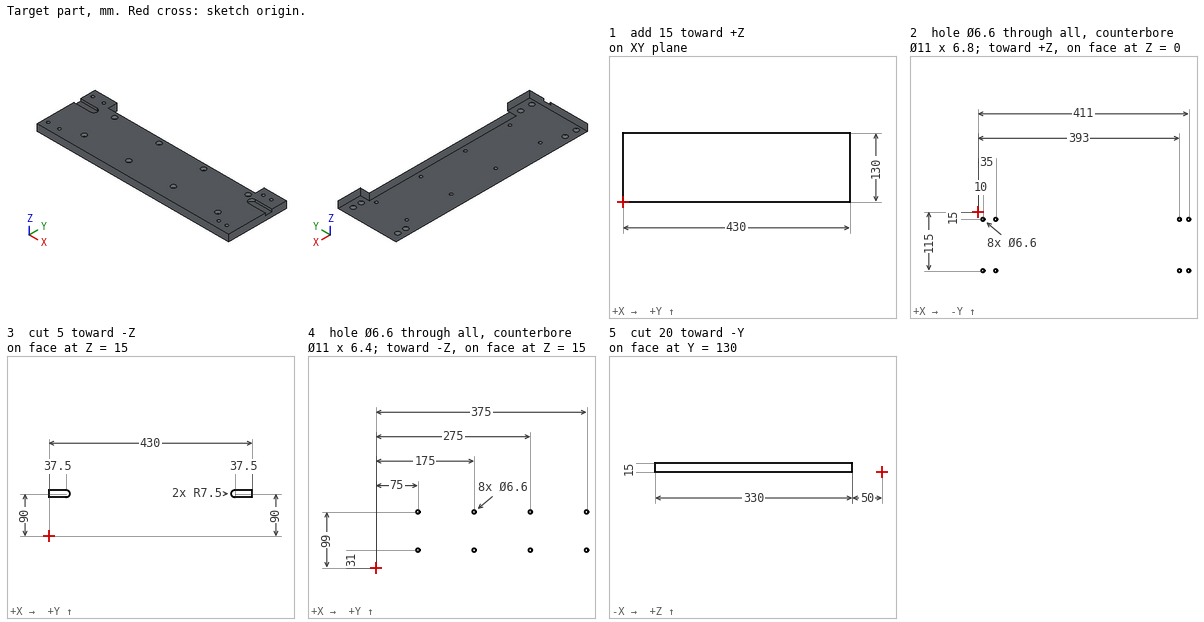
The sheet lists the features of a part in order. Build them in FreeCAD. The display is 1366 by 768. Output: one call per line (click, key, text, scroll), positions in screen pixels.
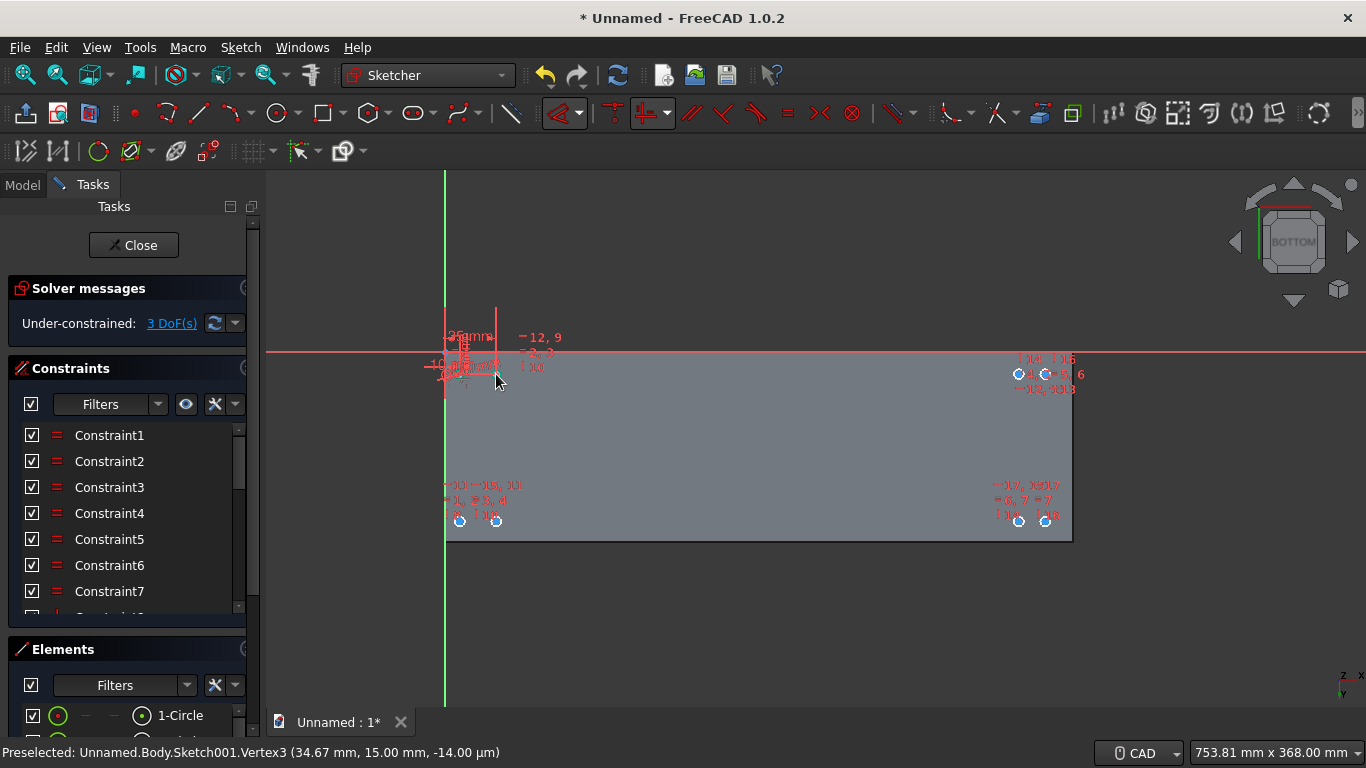
click(460, 522)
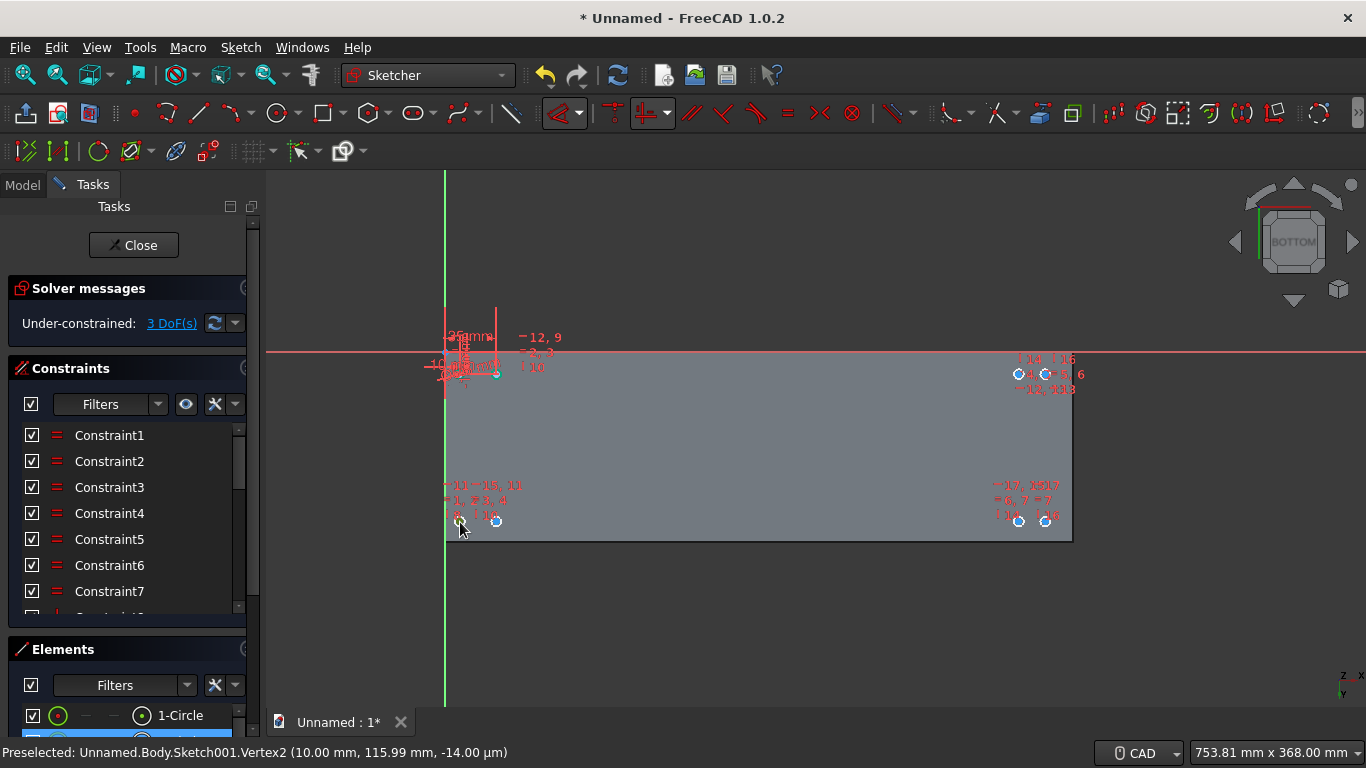
click(582, 114)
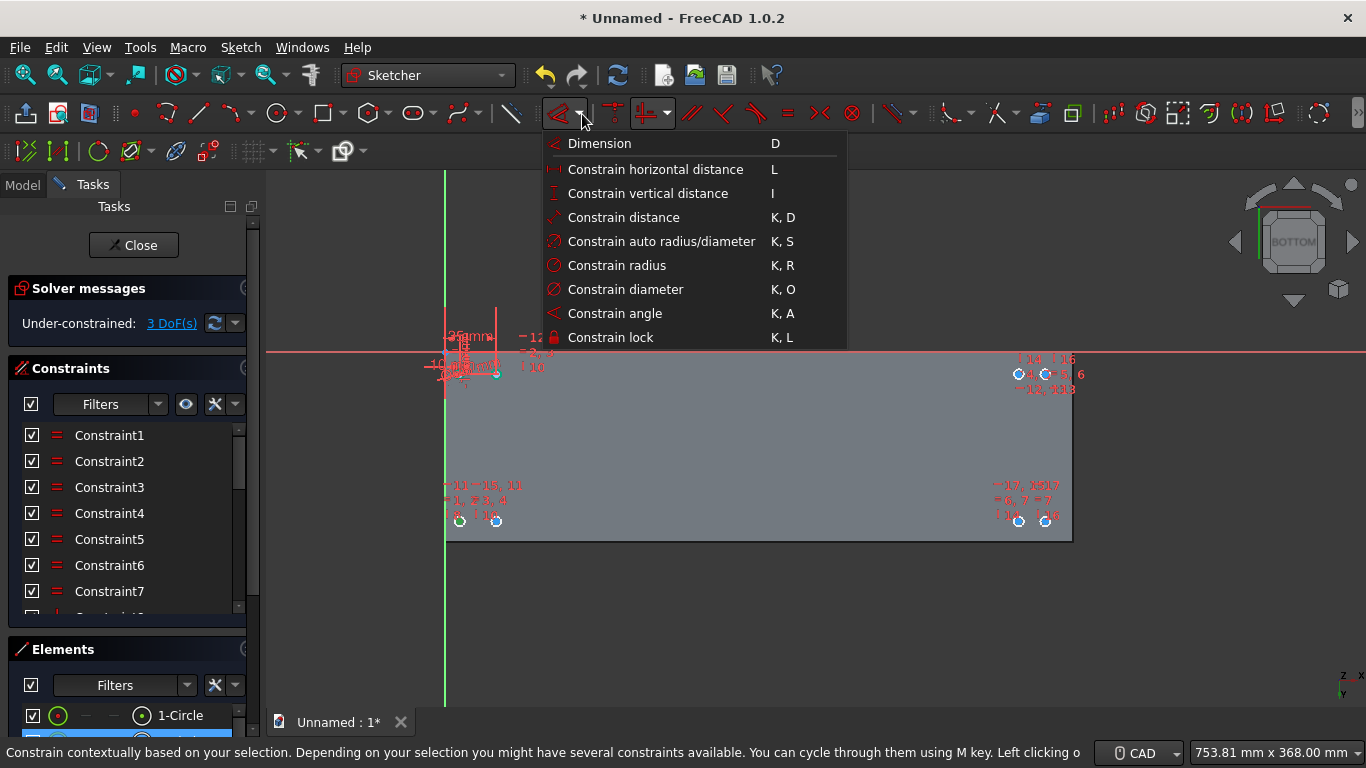
click(695, 193)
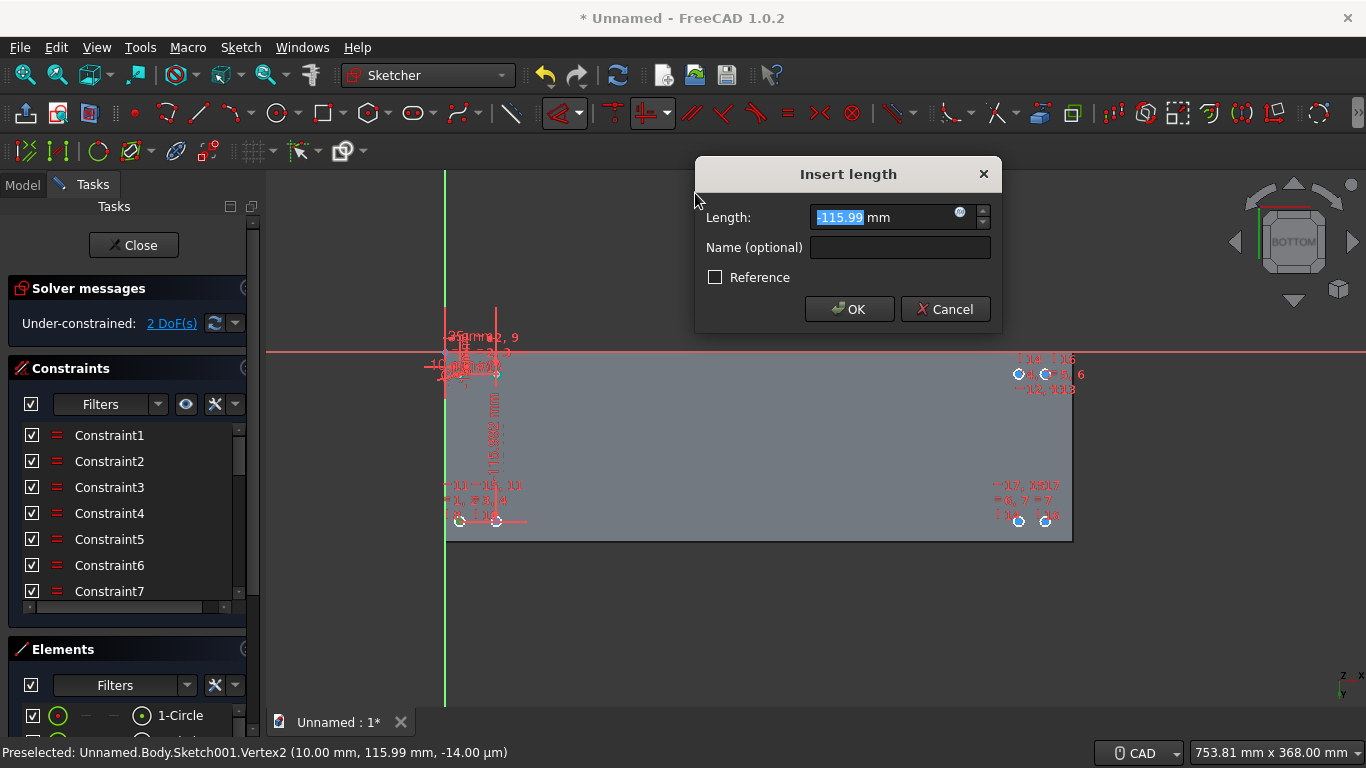
text(-115)
key(Return)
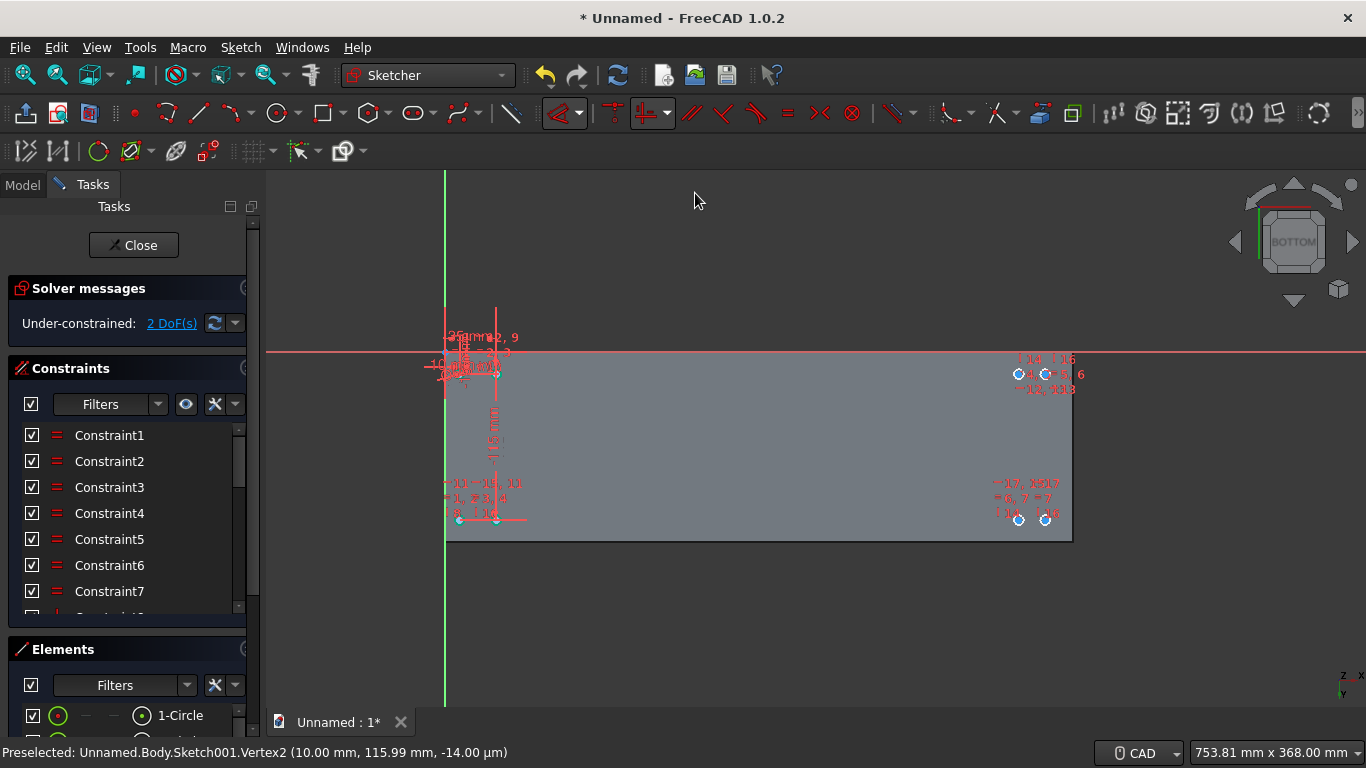
click(1019, 374)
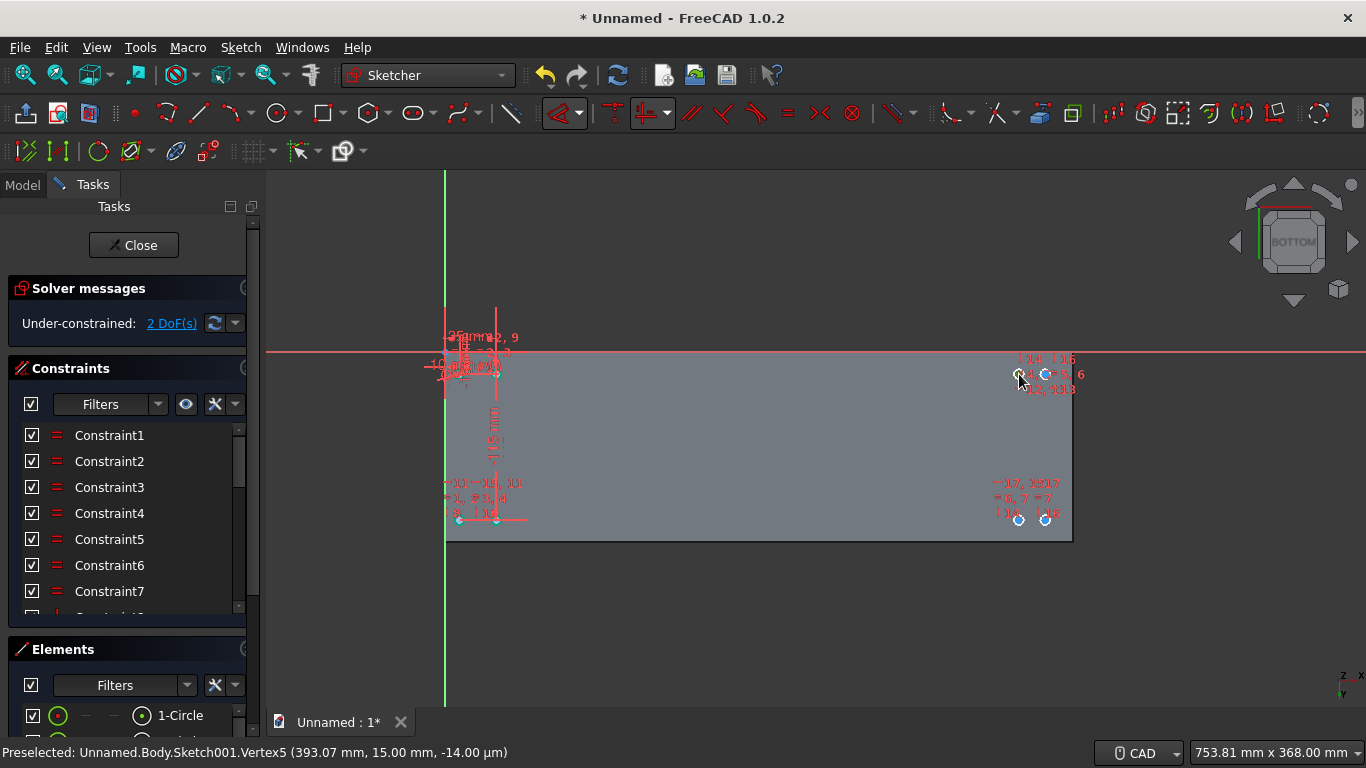
click(582, 114)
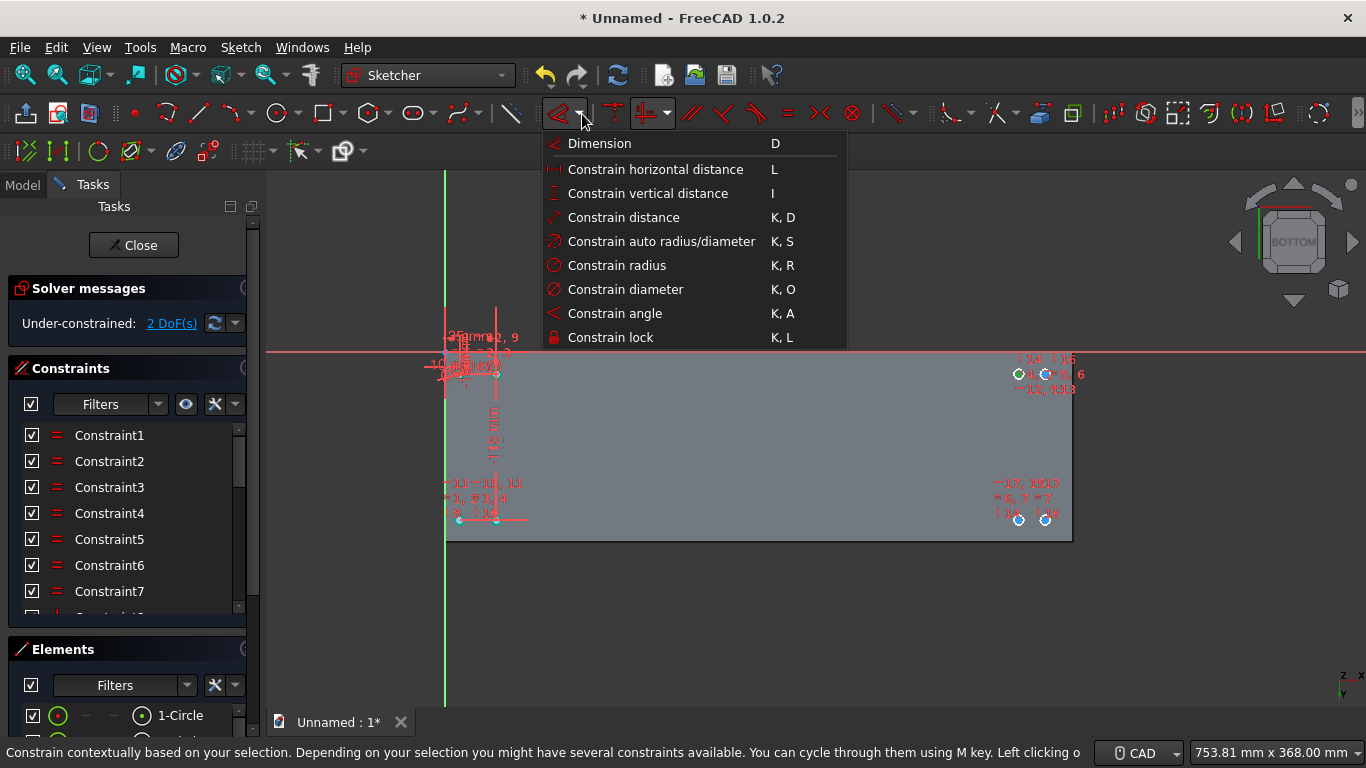
click(695, 169)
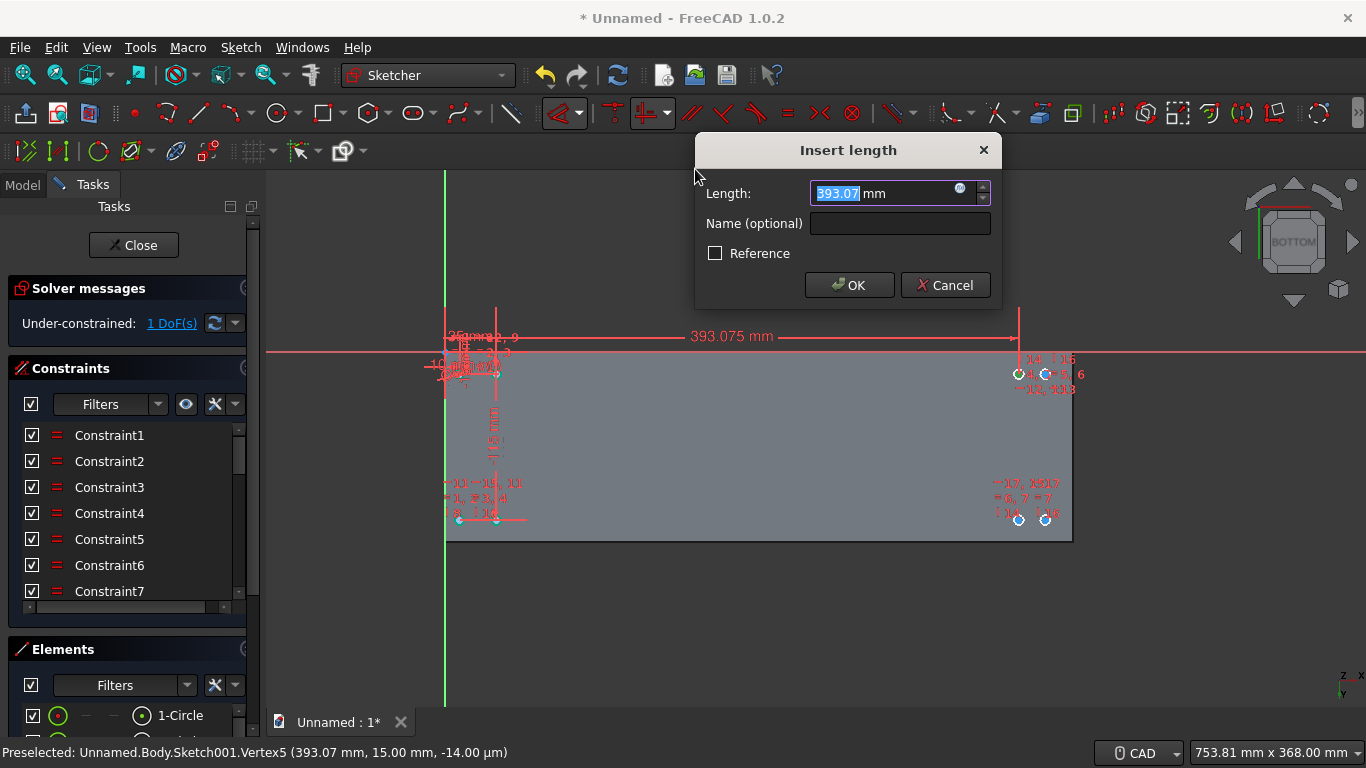
text(393)
key(Return)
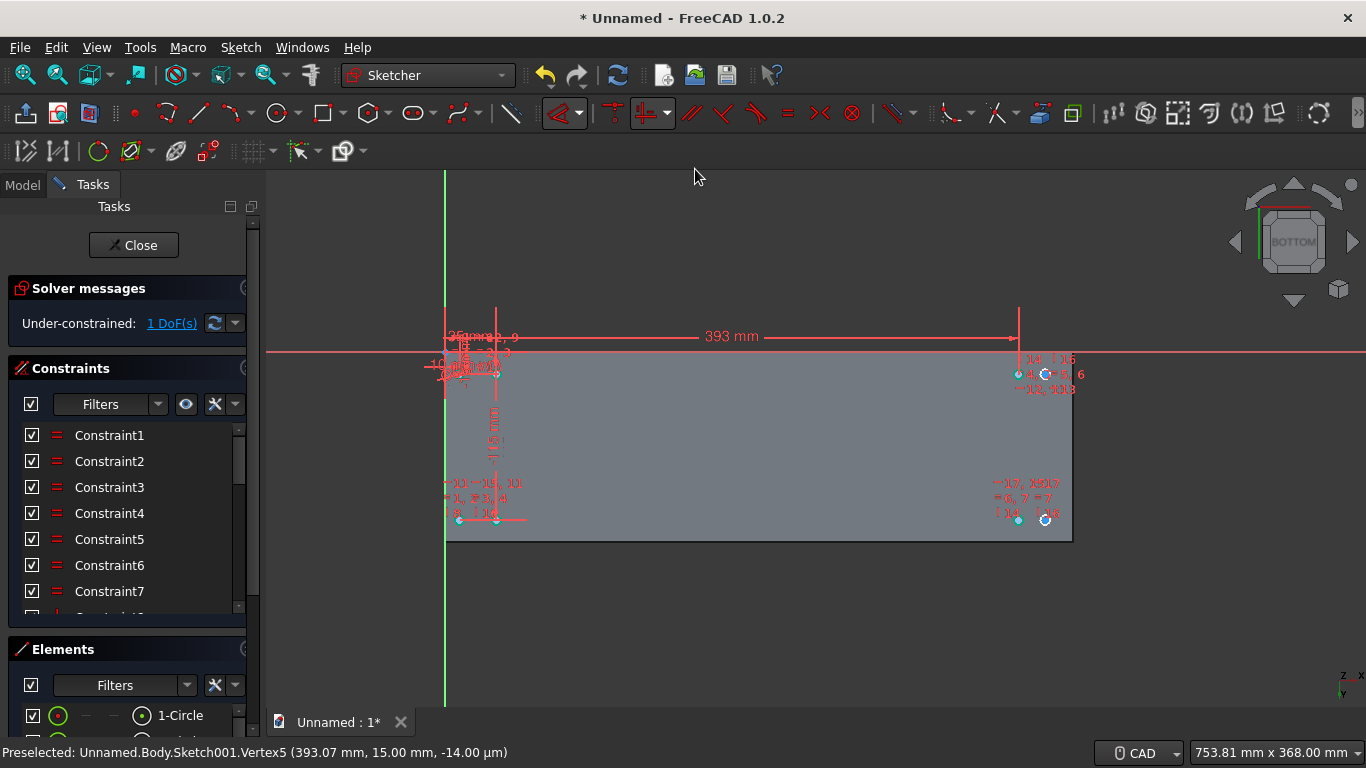
click(1045, 374)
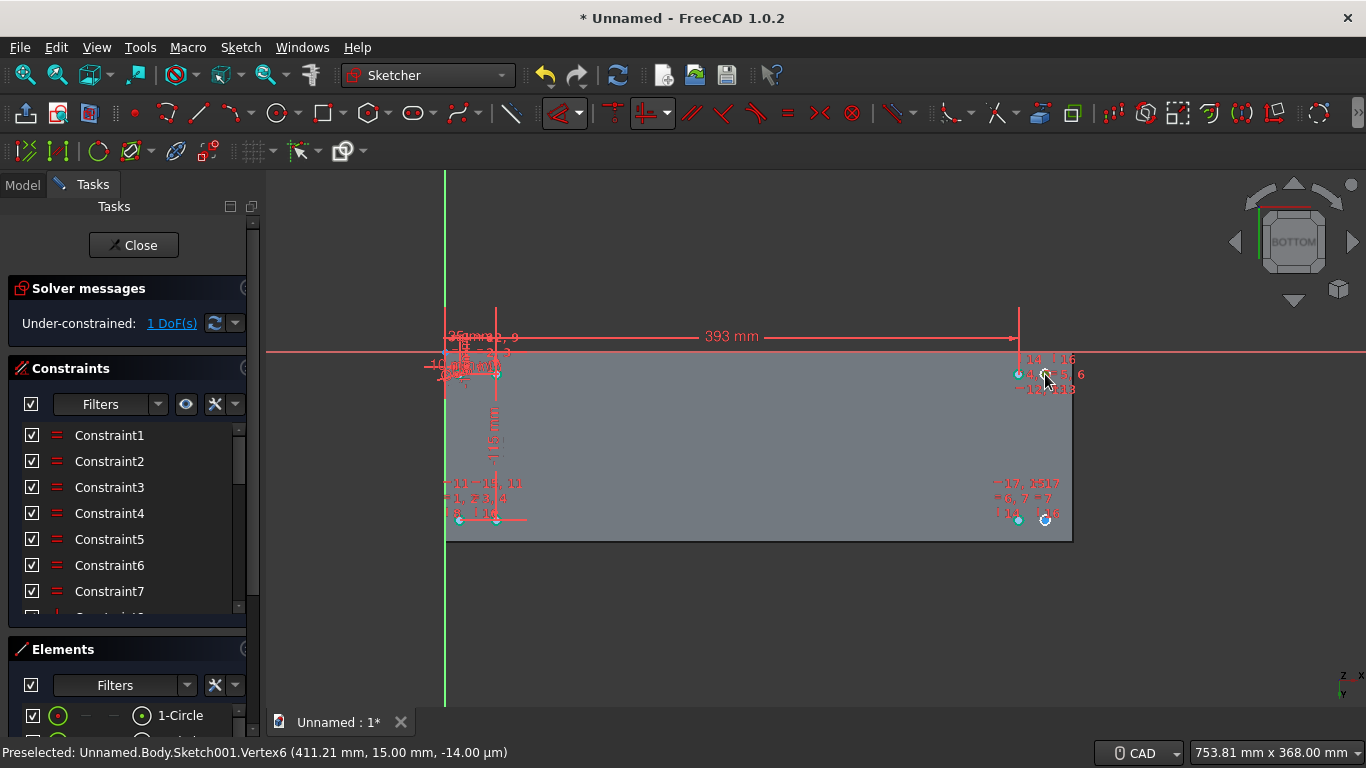
click(582, 114)